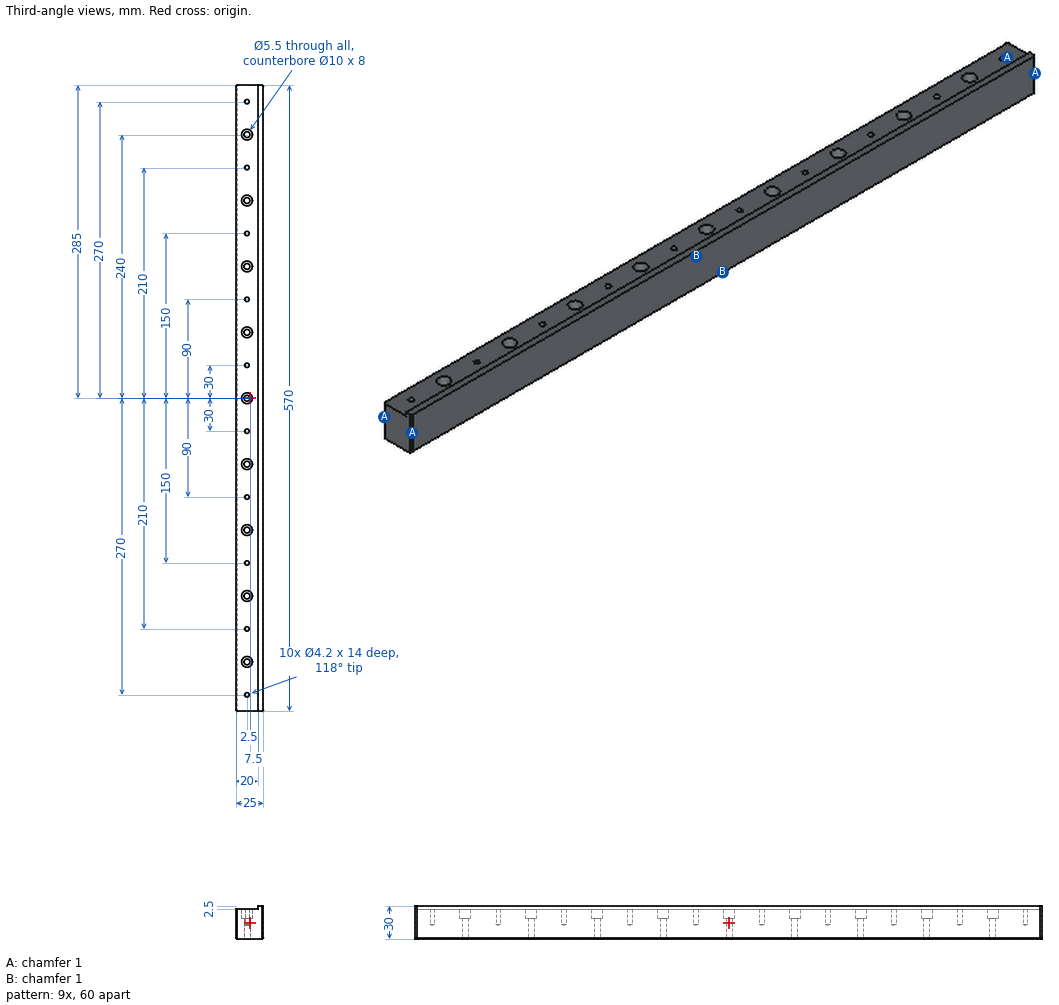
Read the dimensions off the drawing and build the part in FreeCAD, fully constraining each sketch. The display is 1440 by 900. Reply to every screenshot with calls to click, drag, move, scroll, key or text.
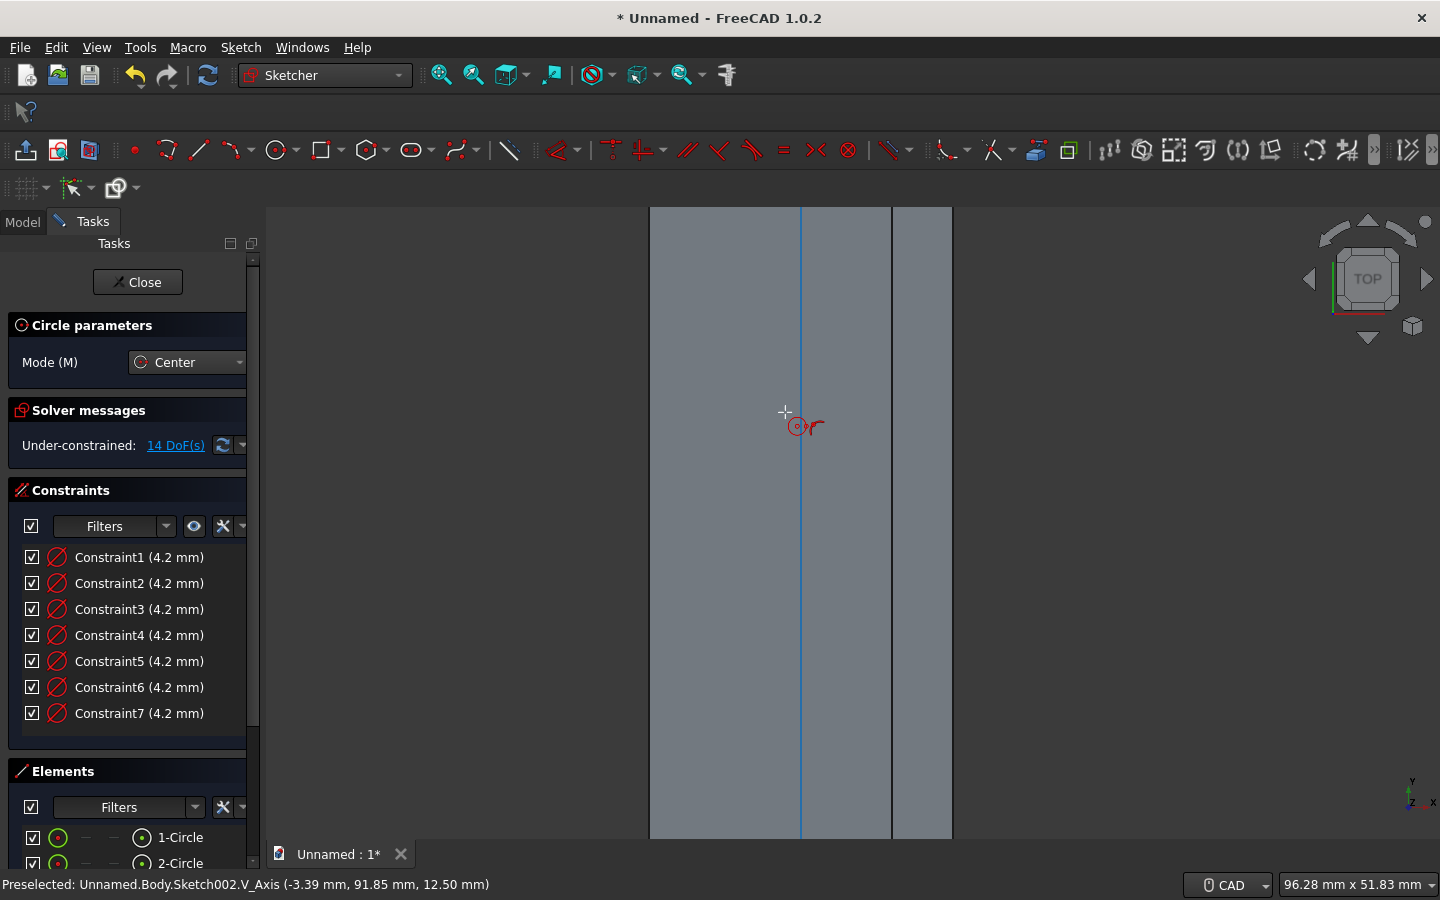
click(771, 403)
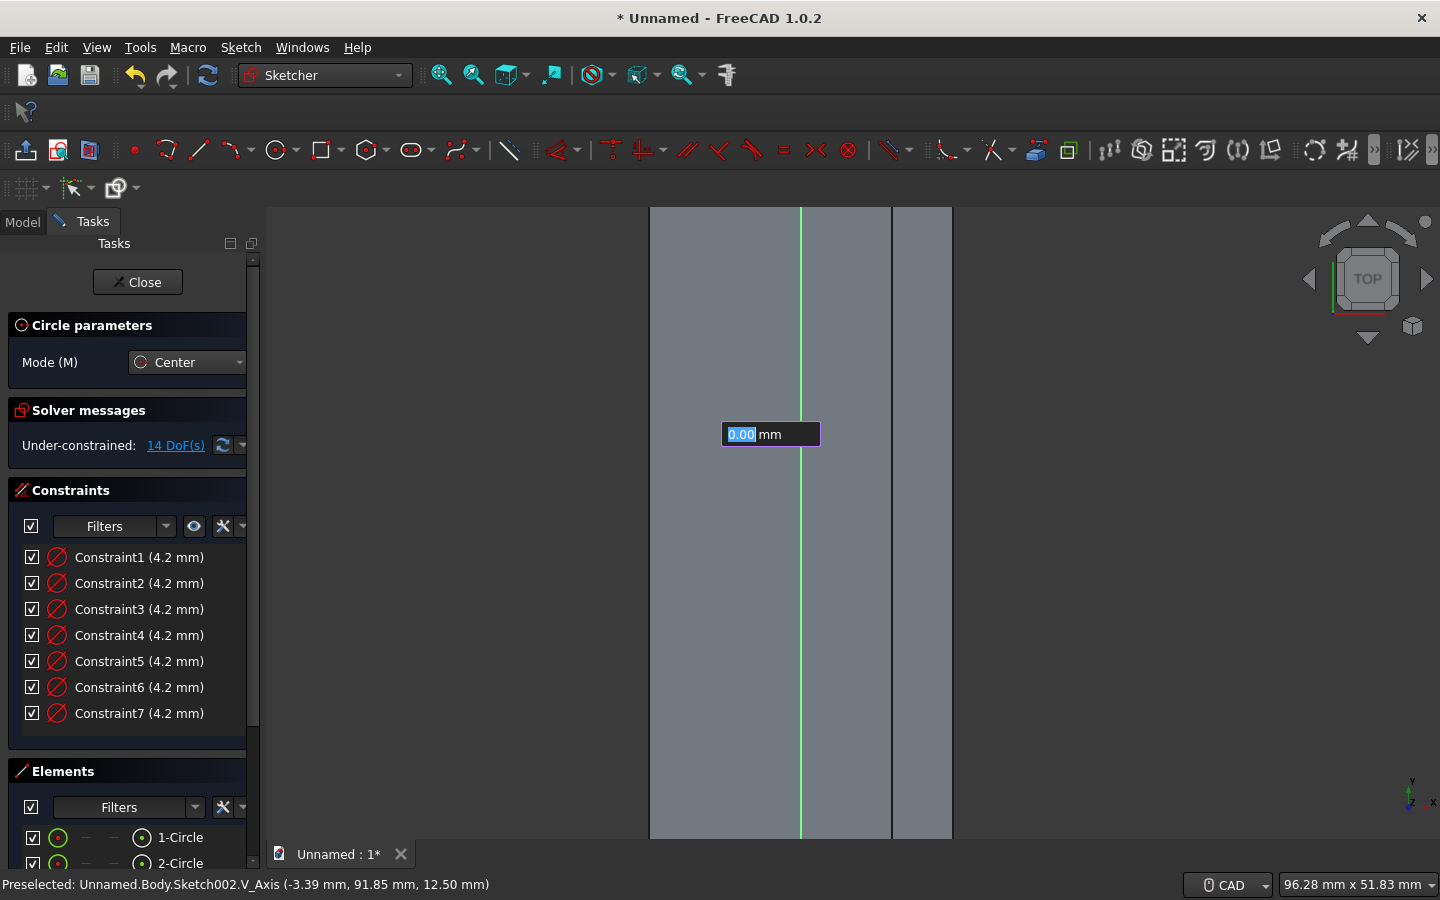
scroll(785, 412, down, 14)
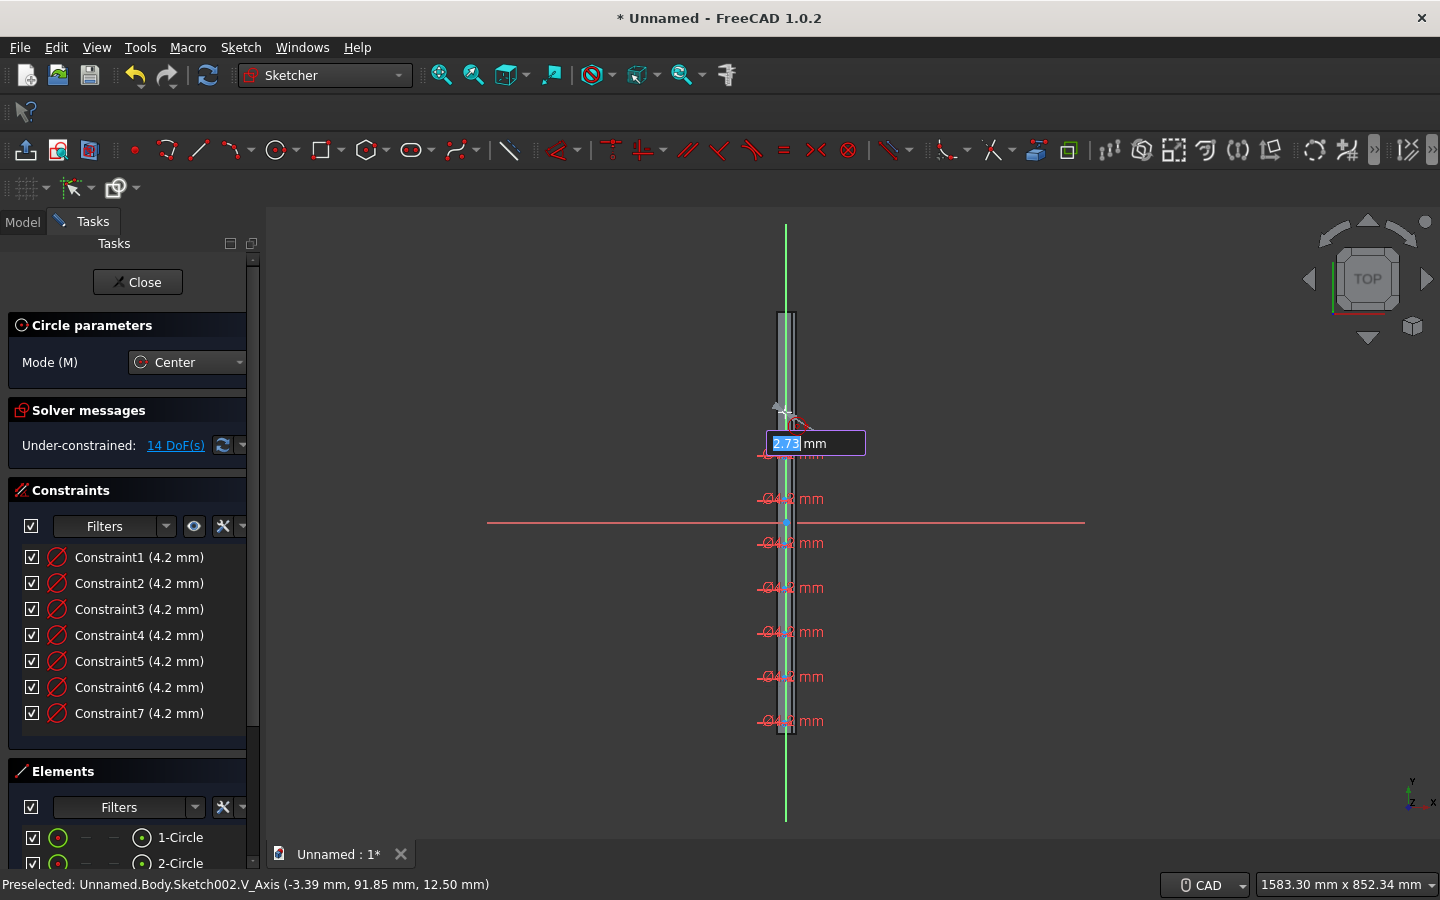
scroll(783, 411, up, 9)
move(783, 407)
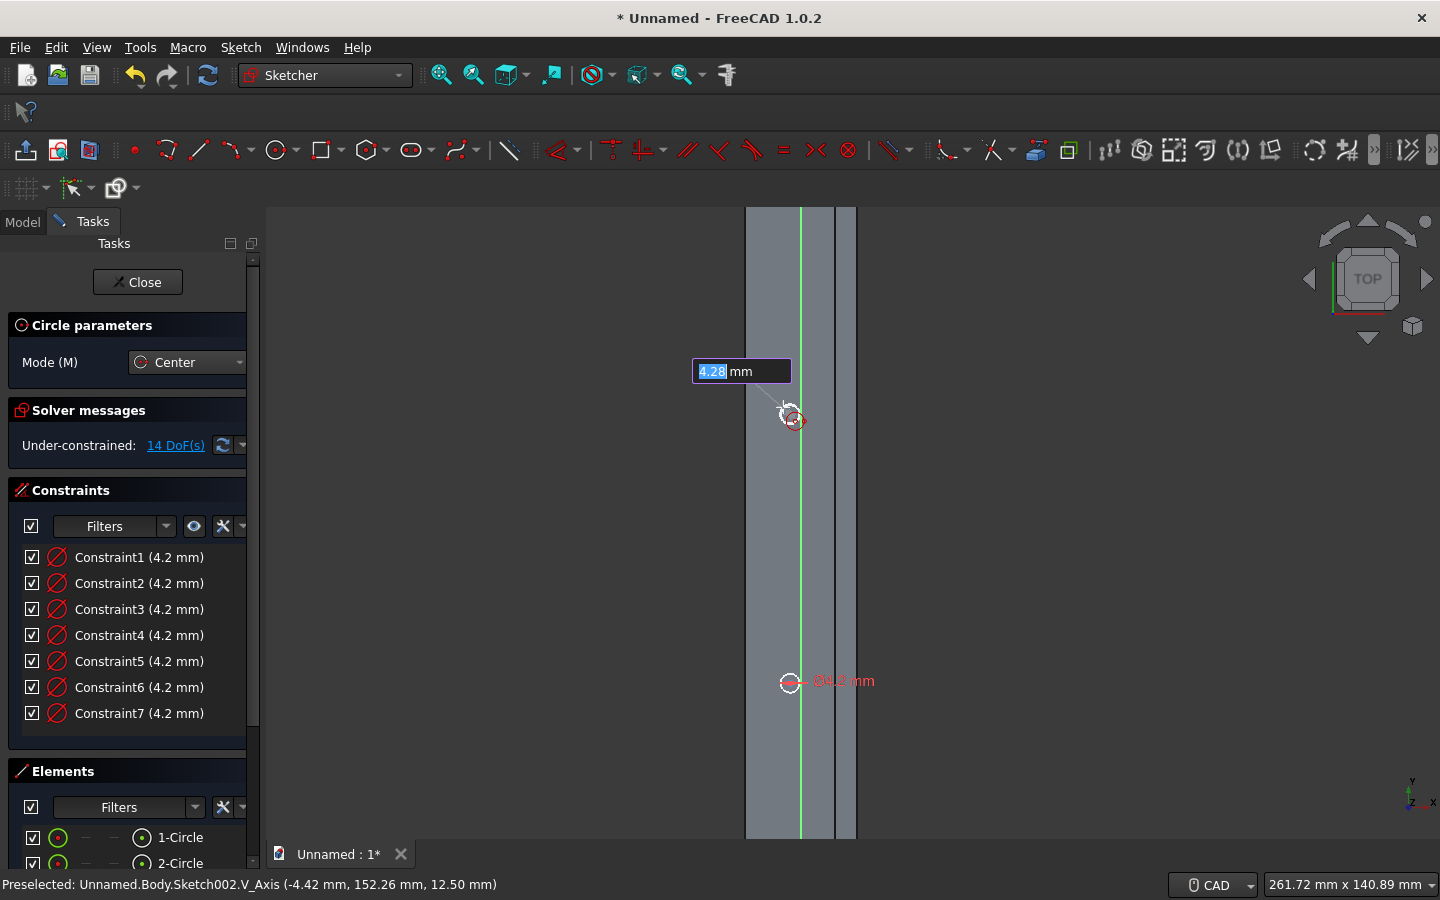
text(4.2)
key(Return)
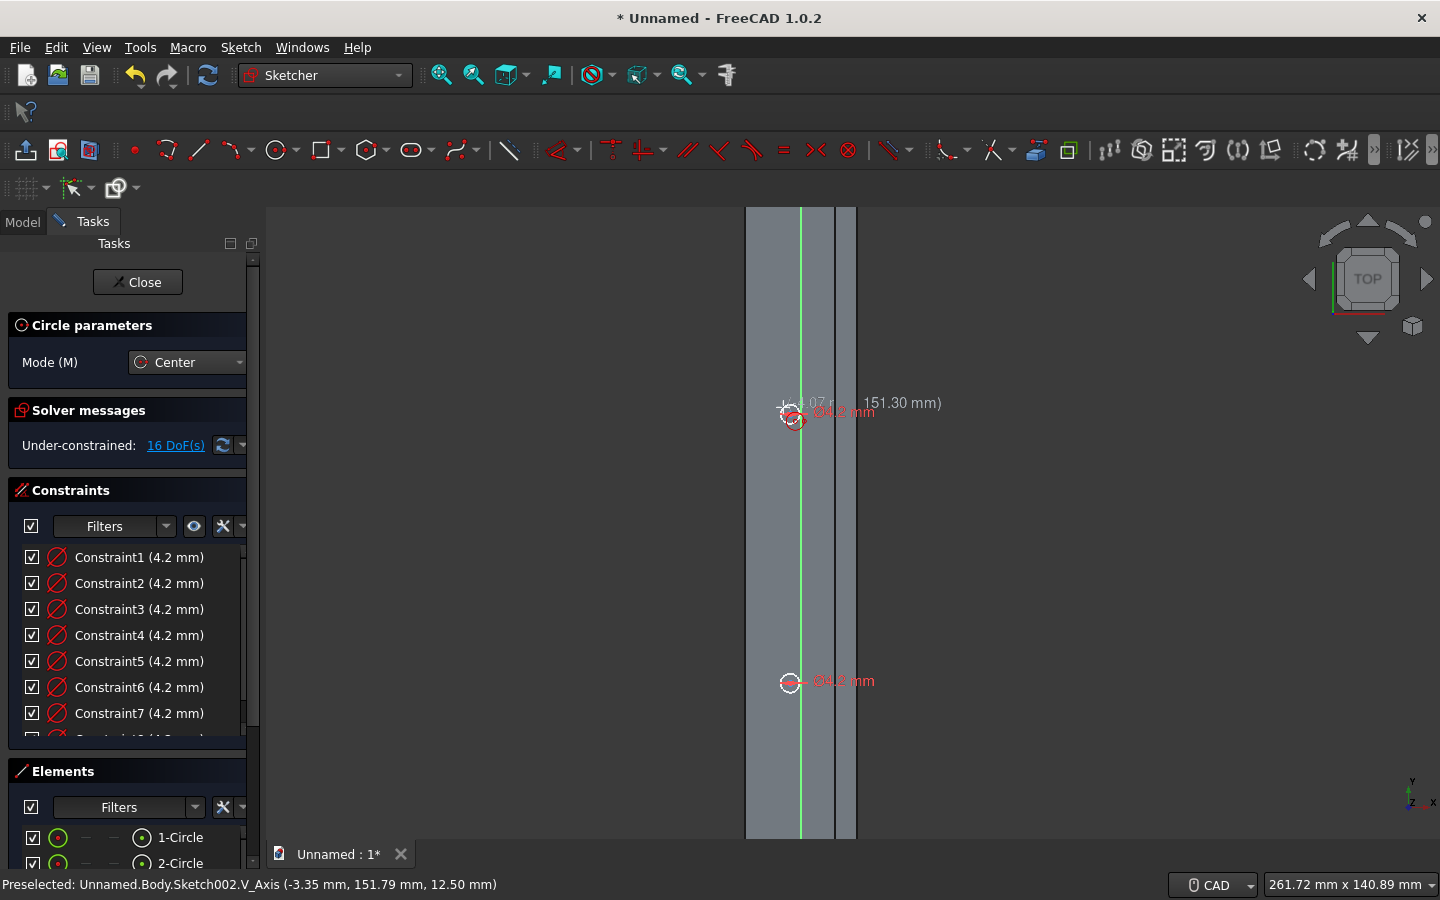
scroll(783, 411, down, 9)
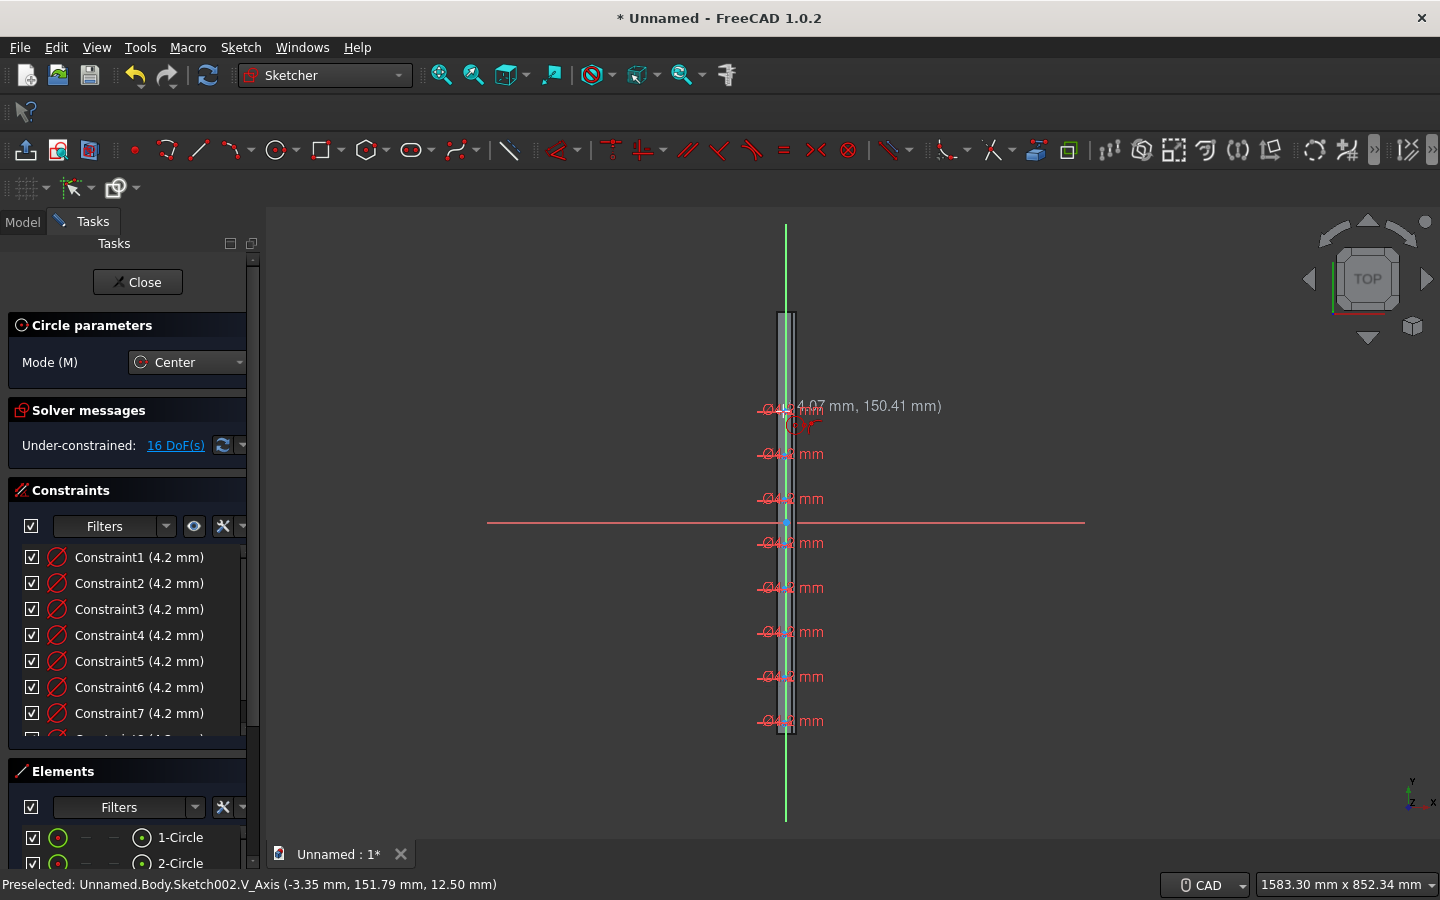
scroll(785, 367, up, 14)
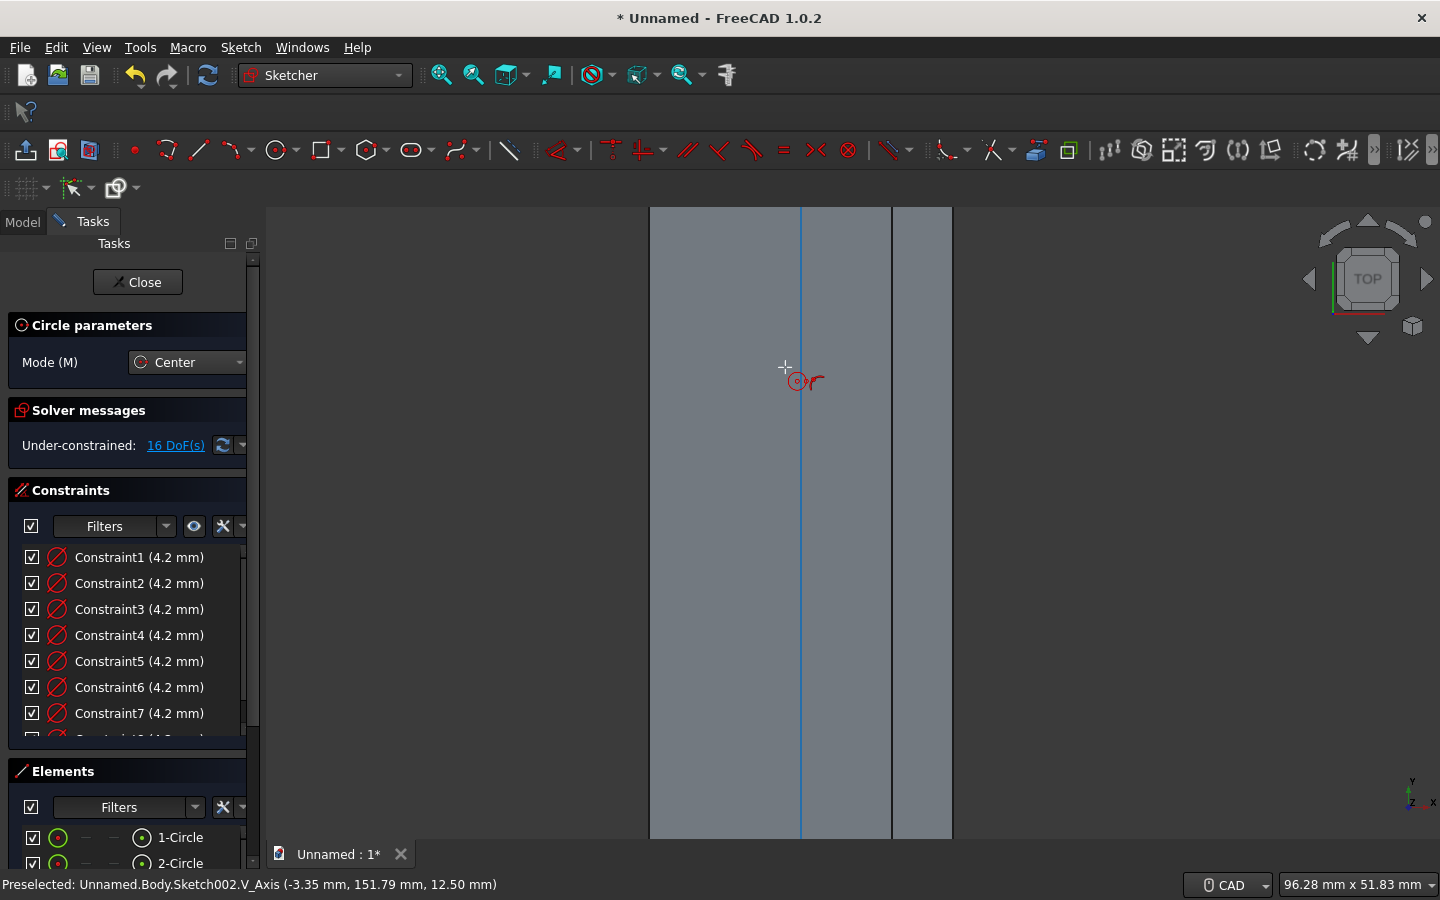
click(771, 367)